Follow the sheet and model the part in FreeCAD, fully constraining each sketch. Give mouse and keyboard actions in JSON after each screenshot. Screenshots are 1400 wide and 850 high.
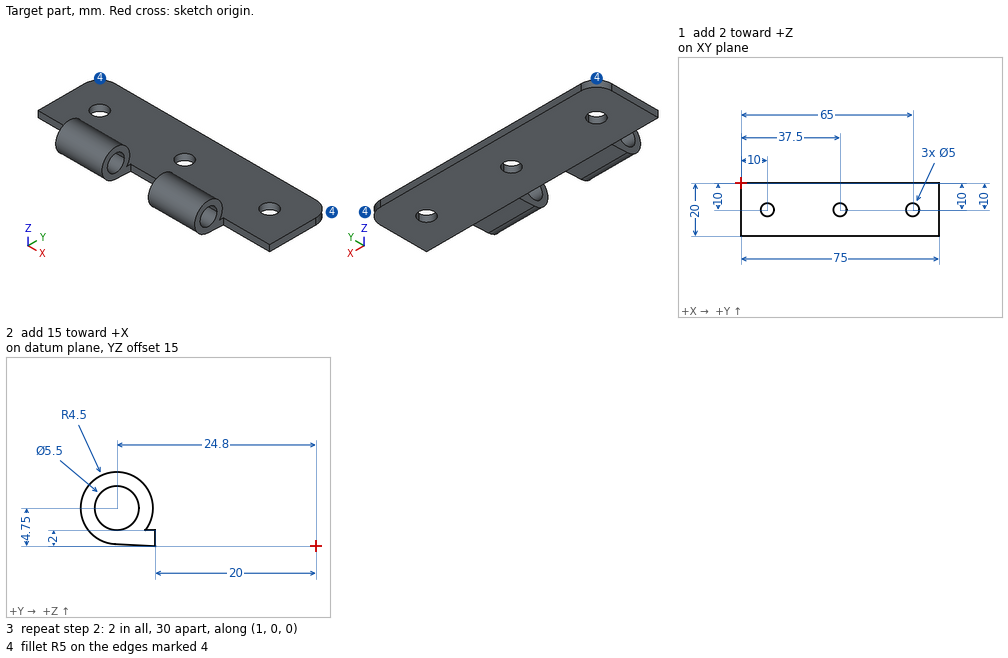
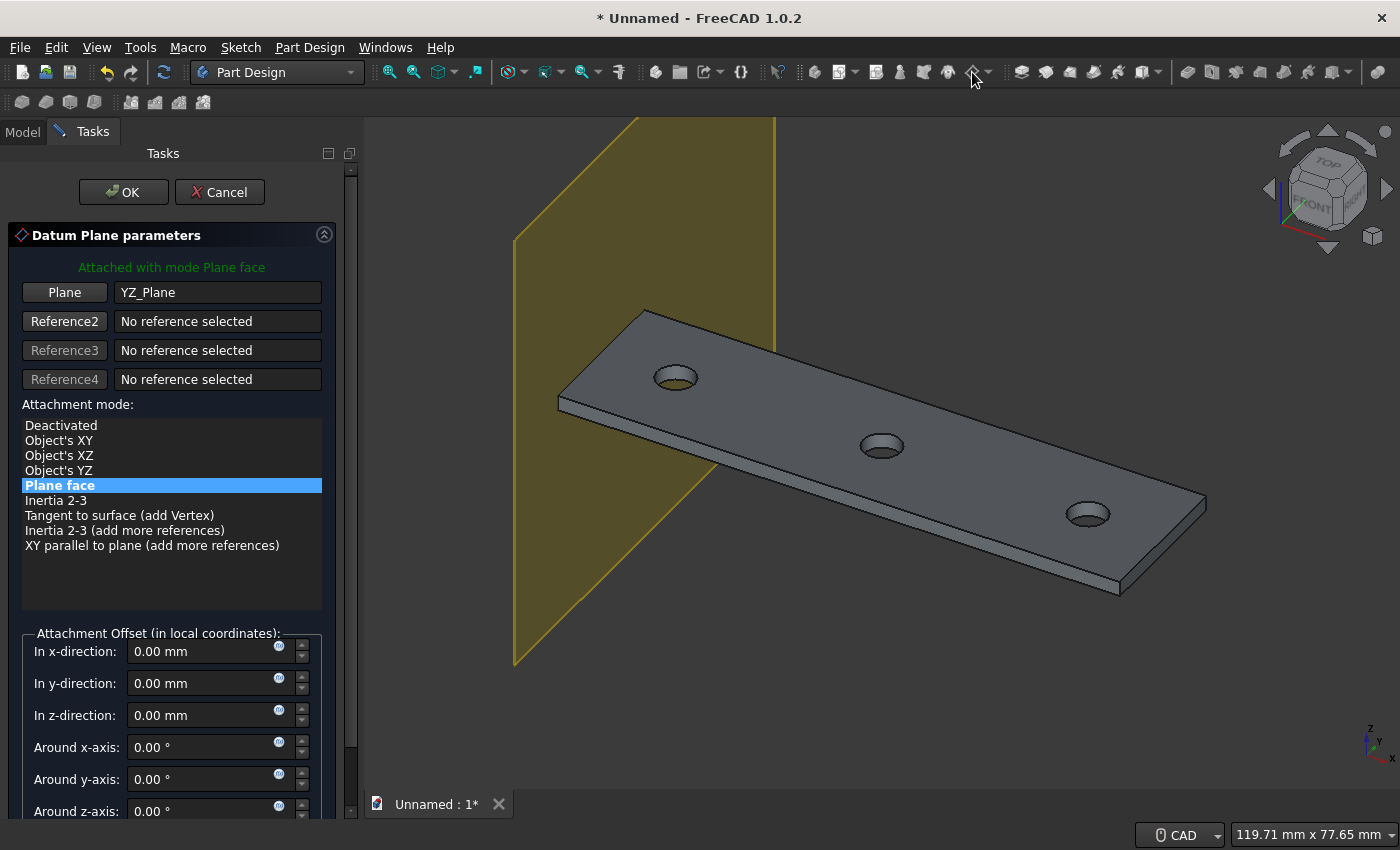
{"action": "triple_click", "coordinate": [210, 715]}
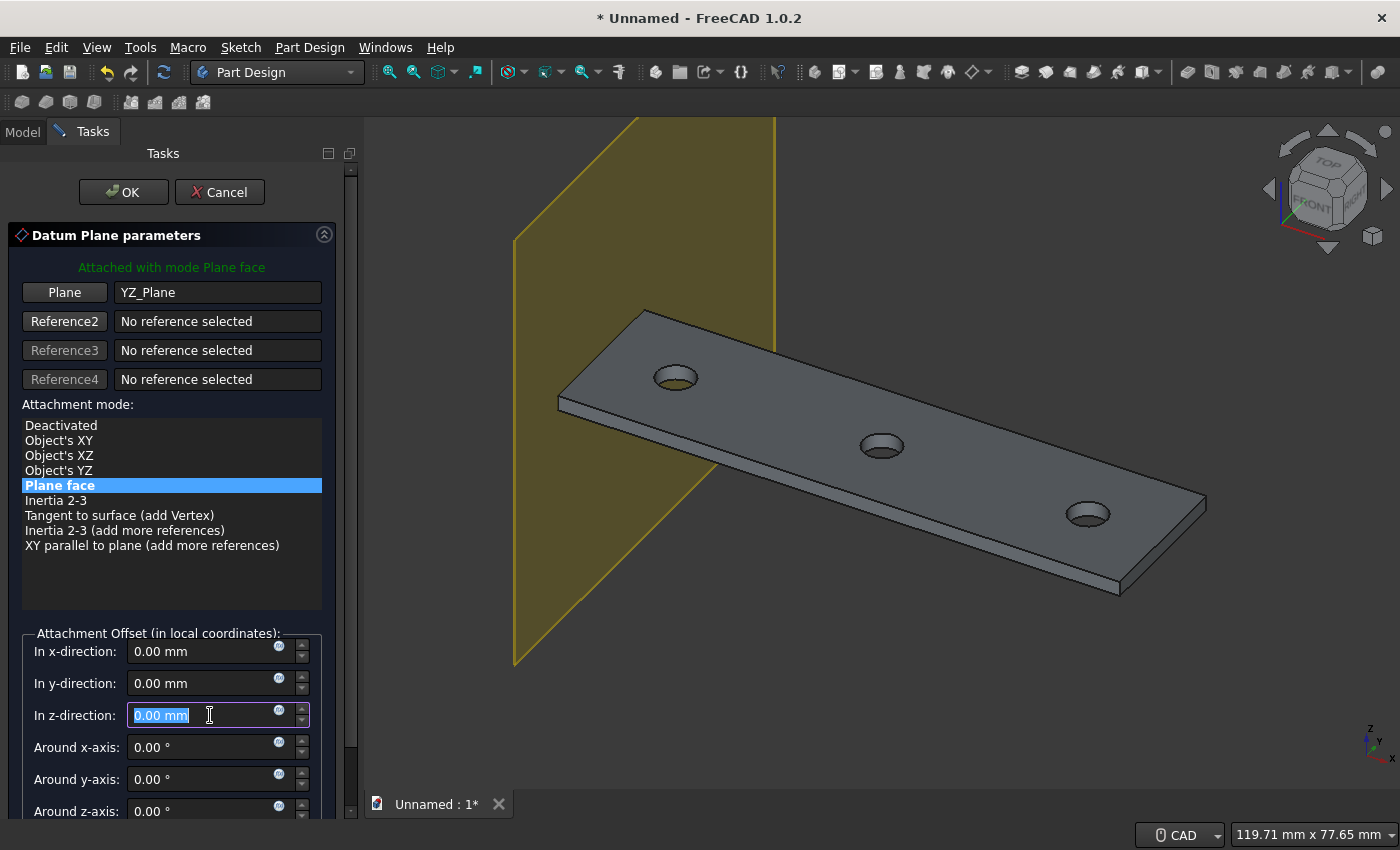
{"action": "type", "text": "15"}
{"action": "key", "text": "Tab"}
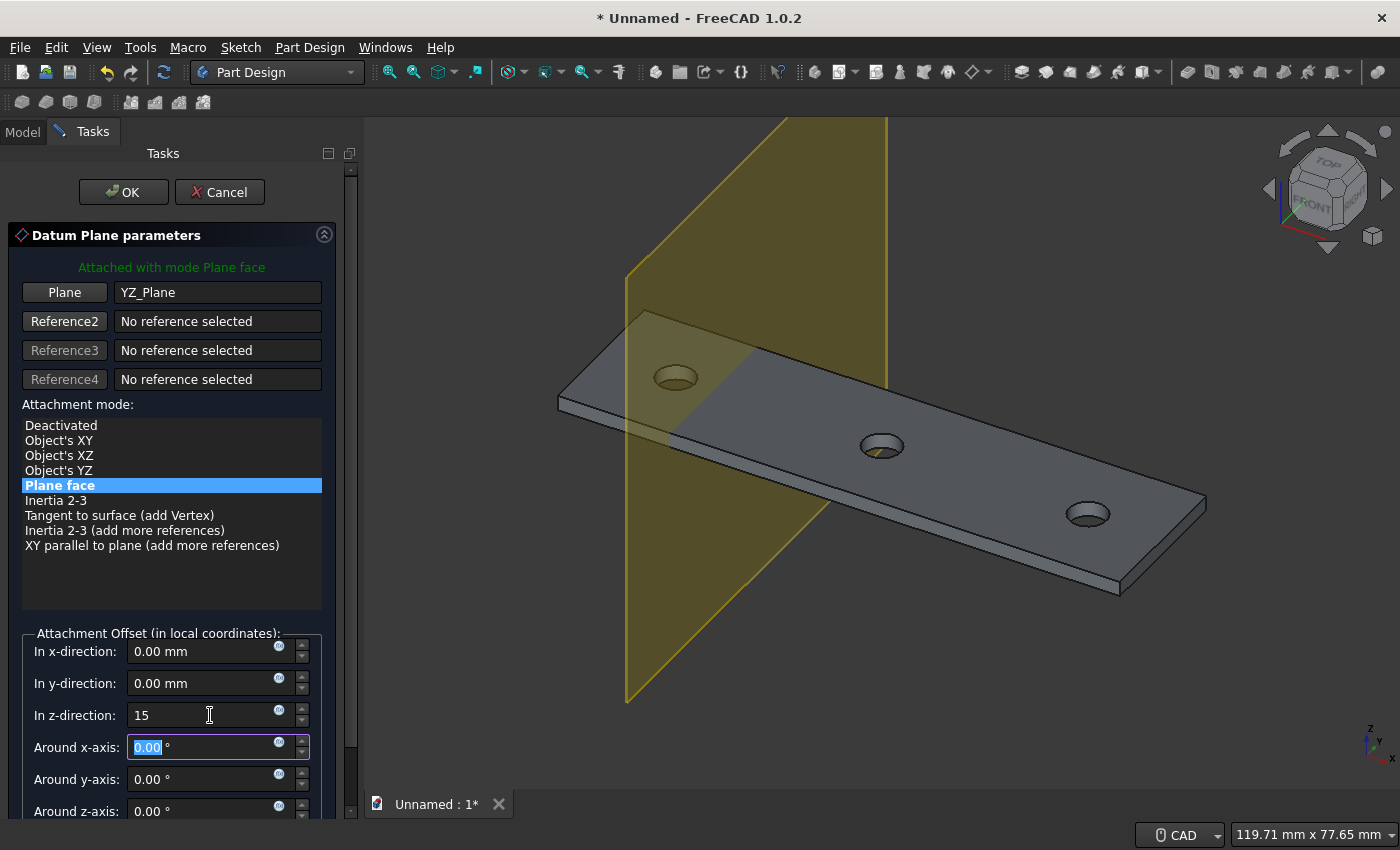
{"action": "left_click", "coordinate": [124, 192]}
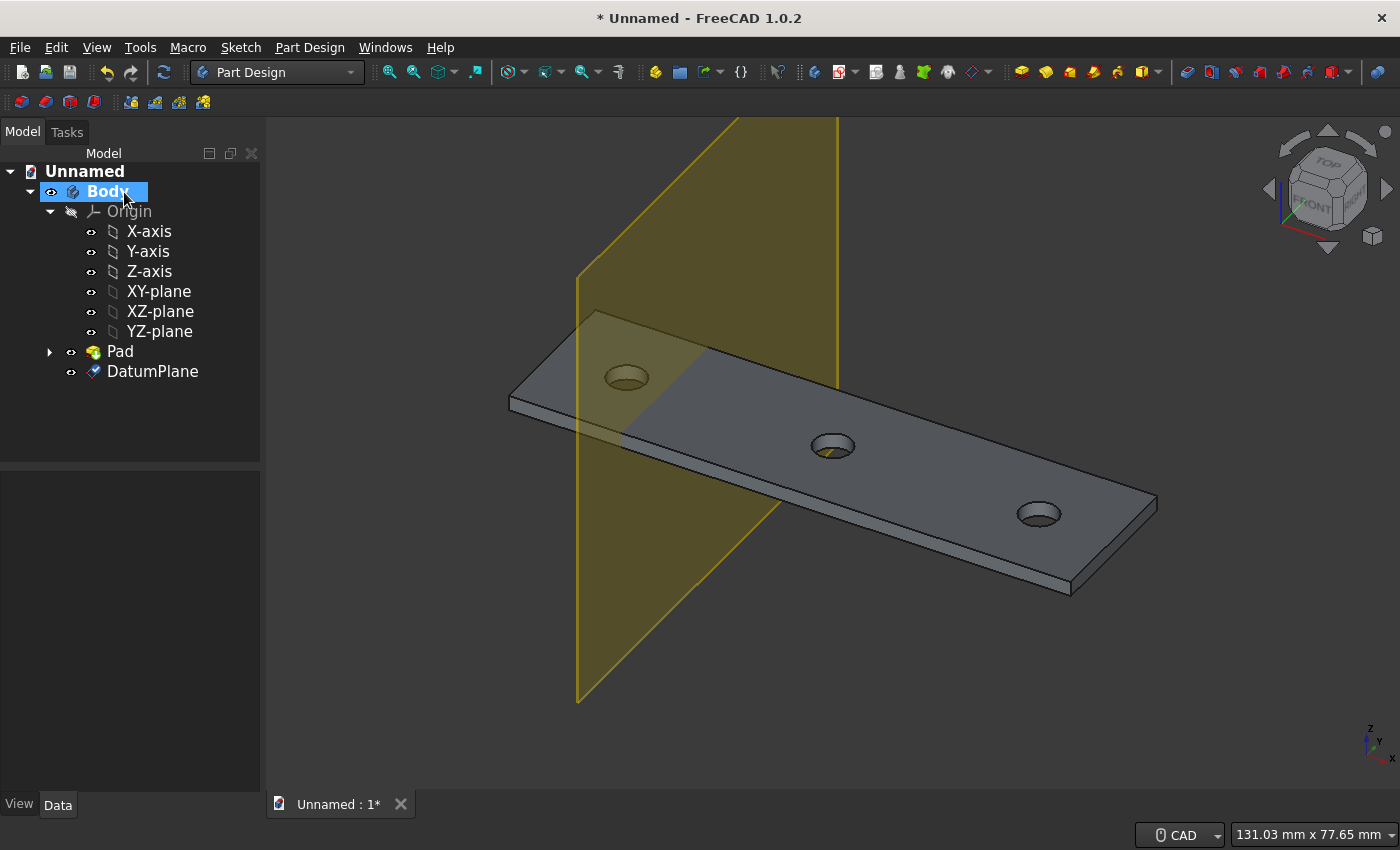
{"action": "left_click", "coordinate": [116, 372]}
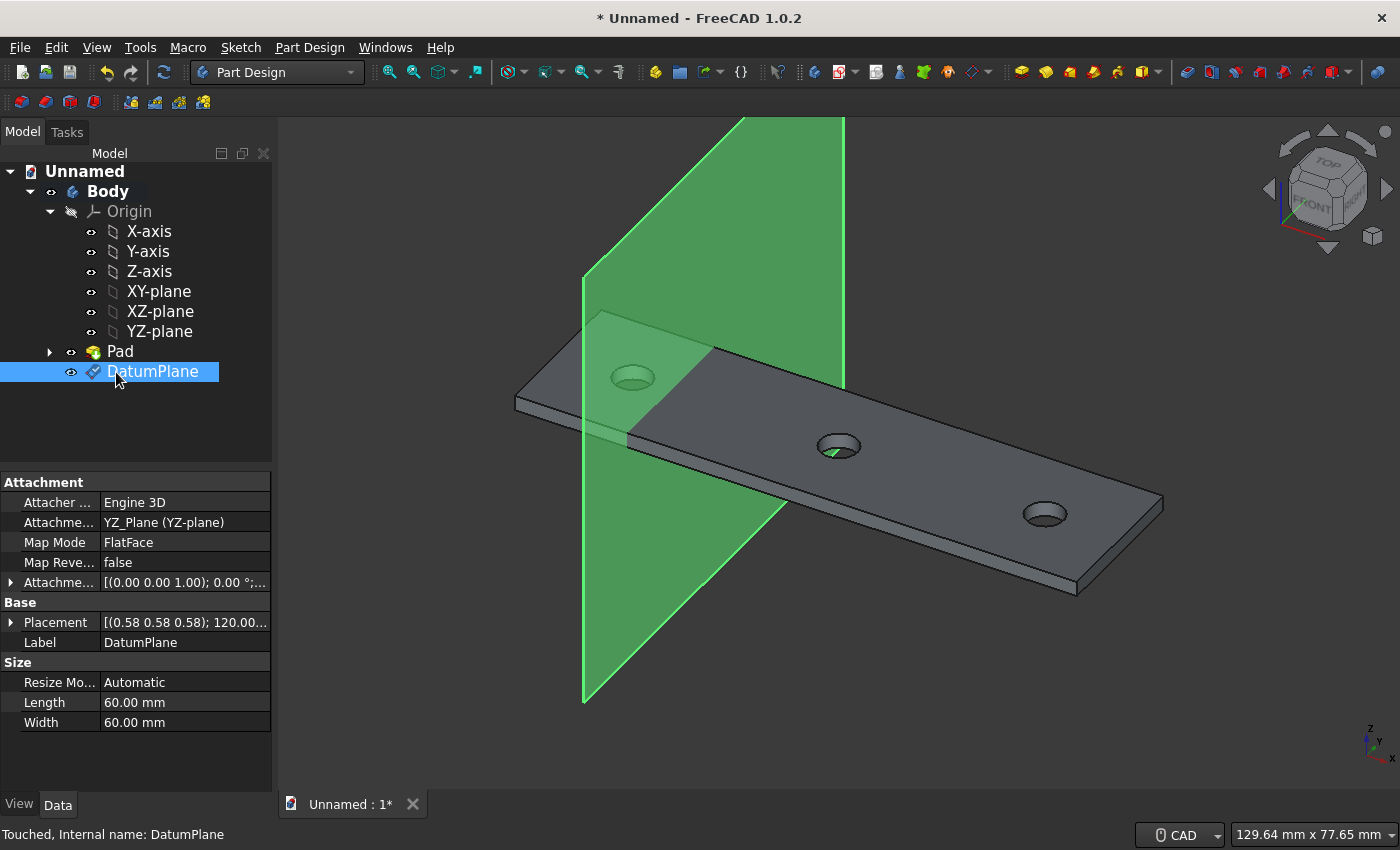
{"action": "left_click", "coordinate": [840, 72]}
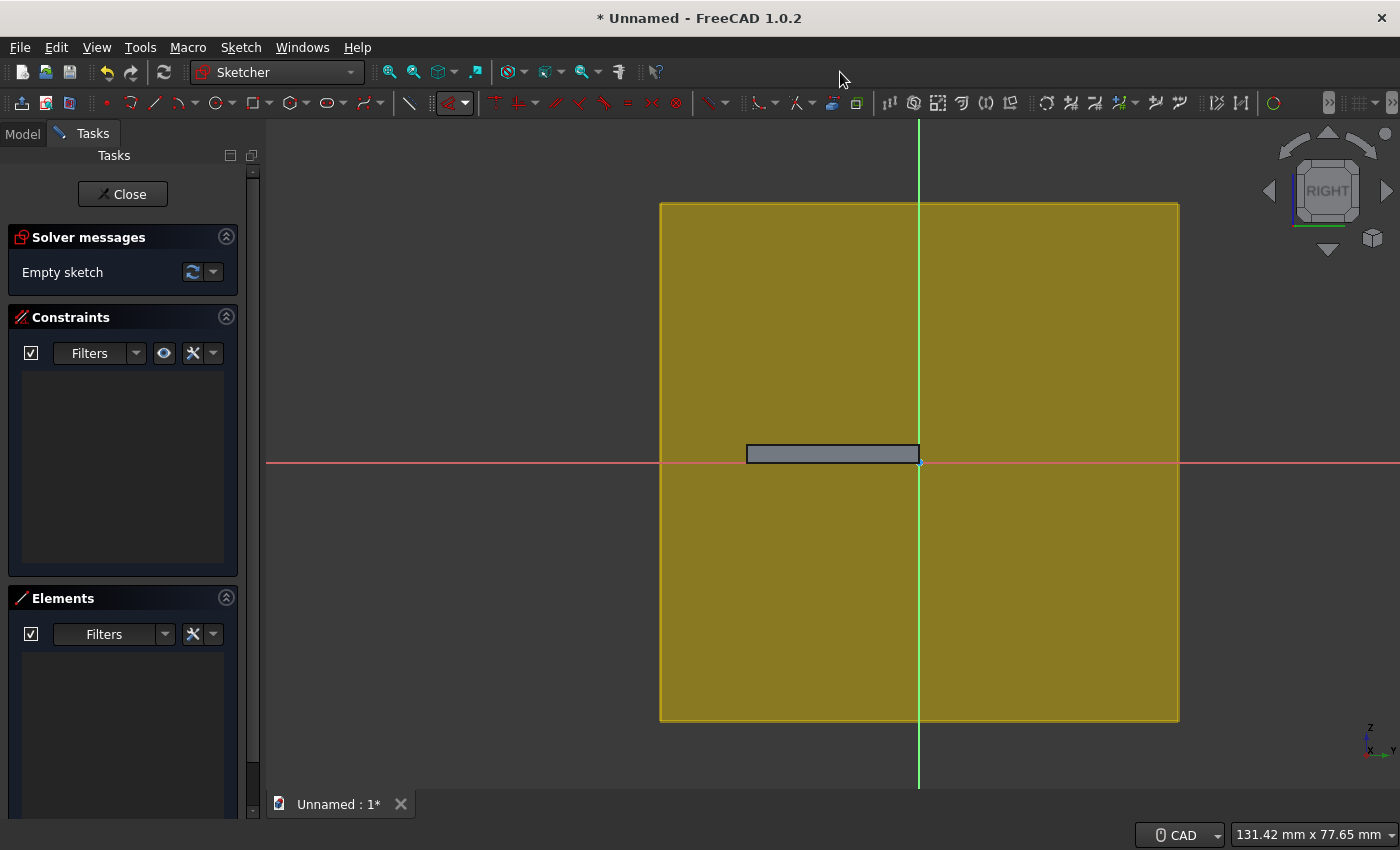
{"action": "key", "text": "q s"}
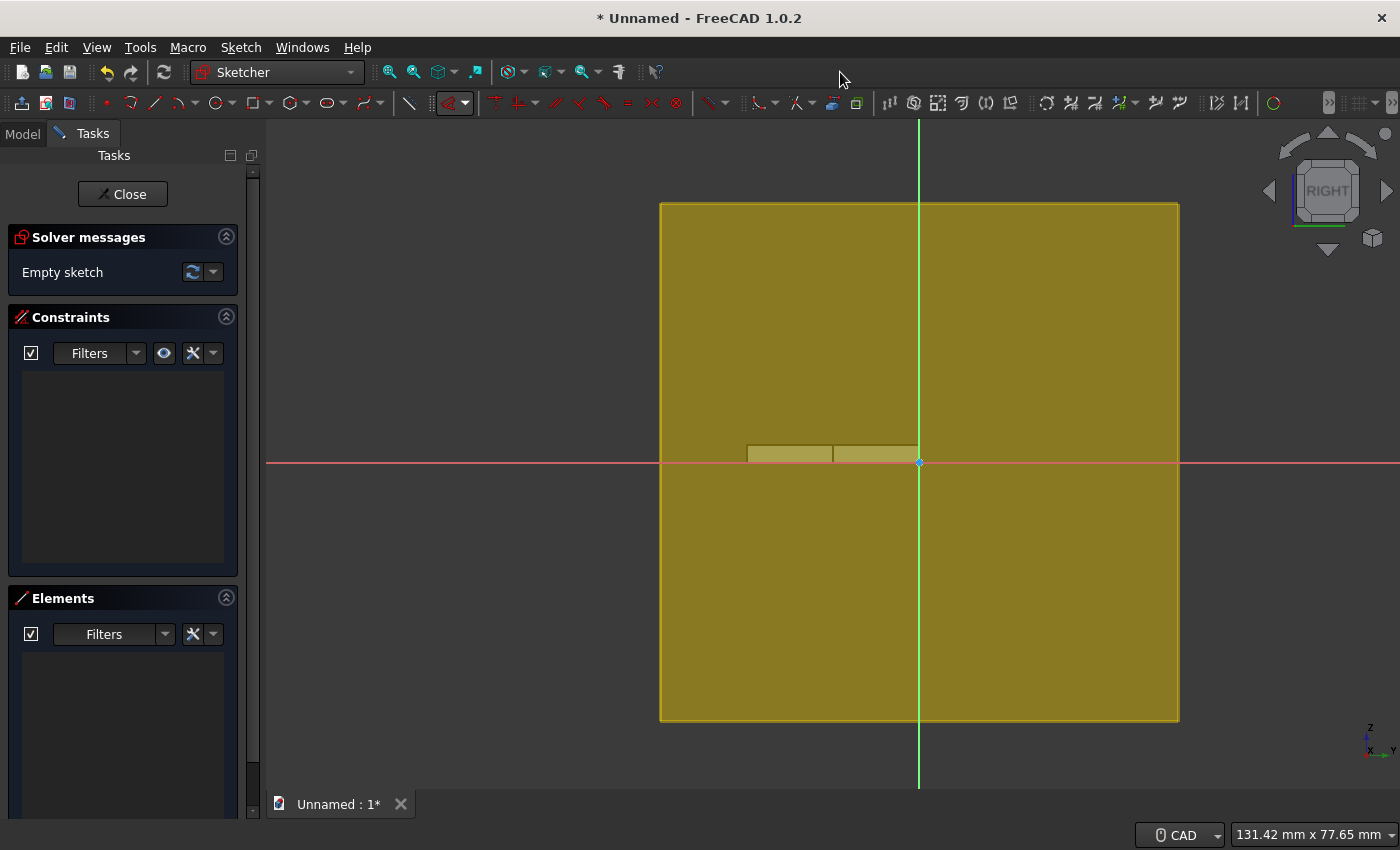
{"action": "scroll", "coordinate": [704, 419], "scroll_direction": "up", "scroll_amount": 9}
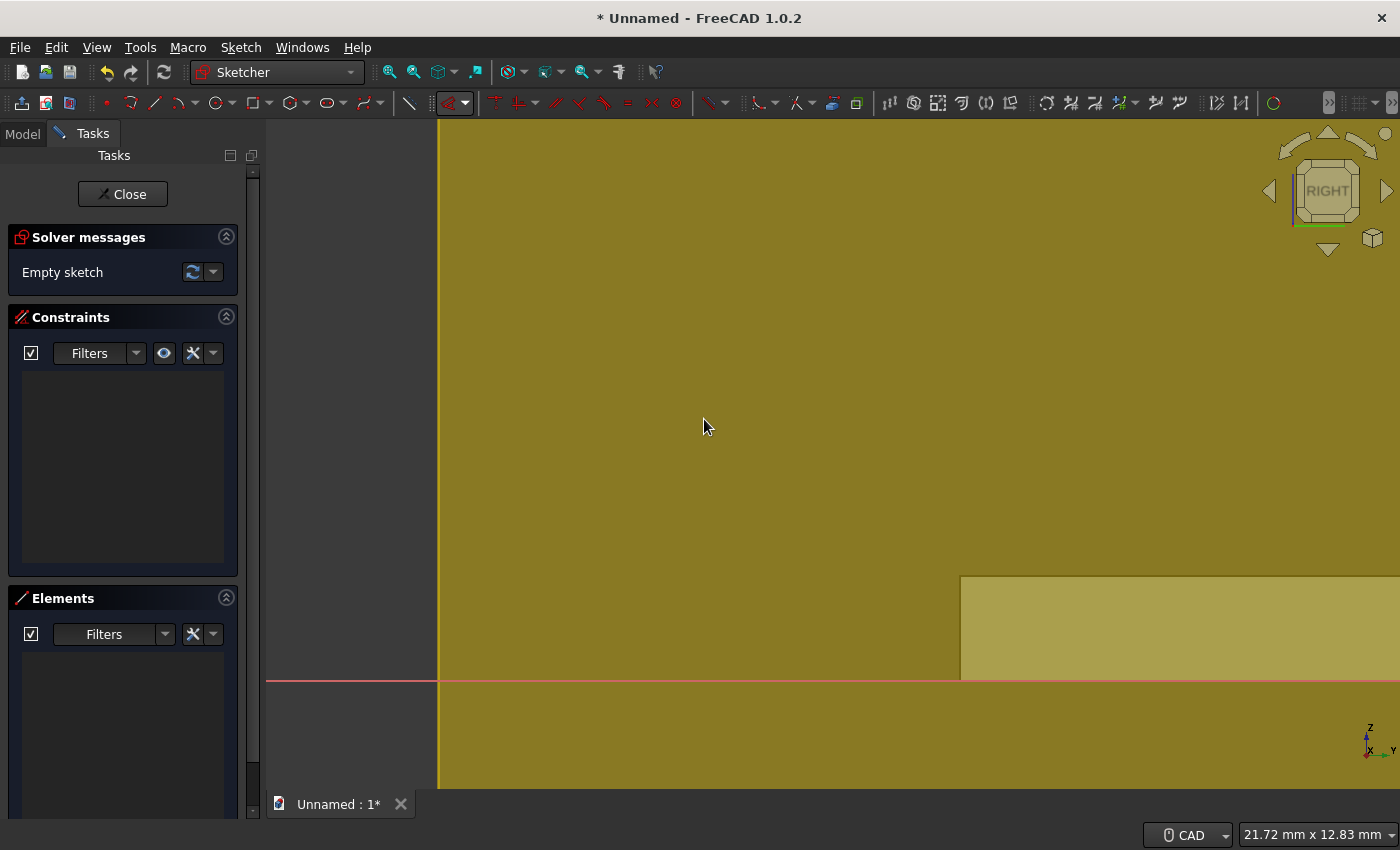
{"action": "key", "text": "g m"}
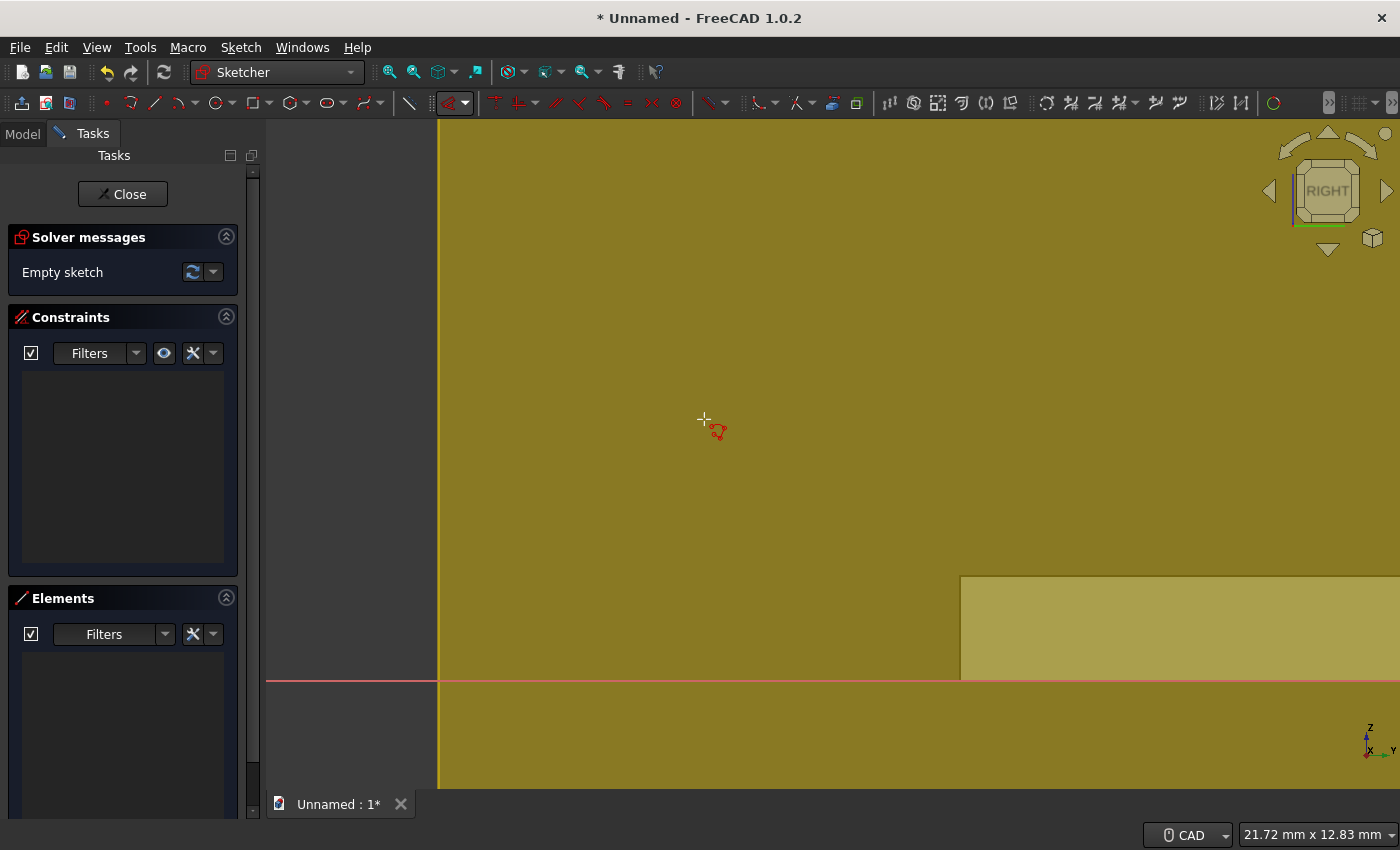
{"action": "left_click", "coordinate": [896, 576]}
{"action": "left_click", "coordinate": [960, 576]}
{"action": "left_click", "coordinate": [960, 681]}
{"action": "left_click", "coordinate": [698, 667]}
{"action": "right_click", "coordinate": [698, 667]}